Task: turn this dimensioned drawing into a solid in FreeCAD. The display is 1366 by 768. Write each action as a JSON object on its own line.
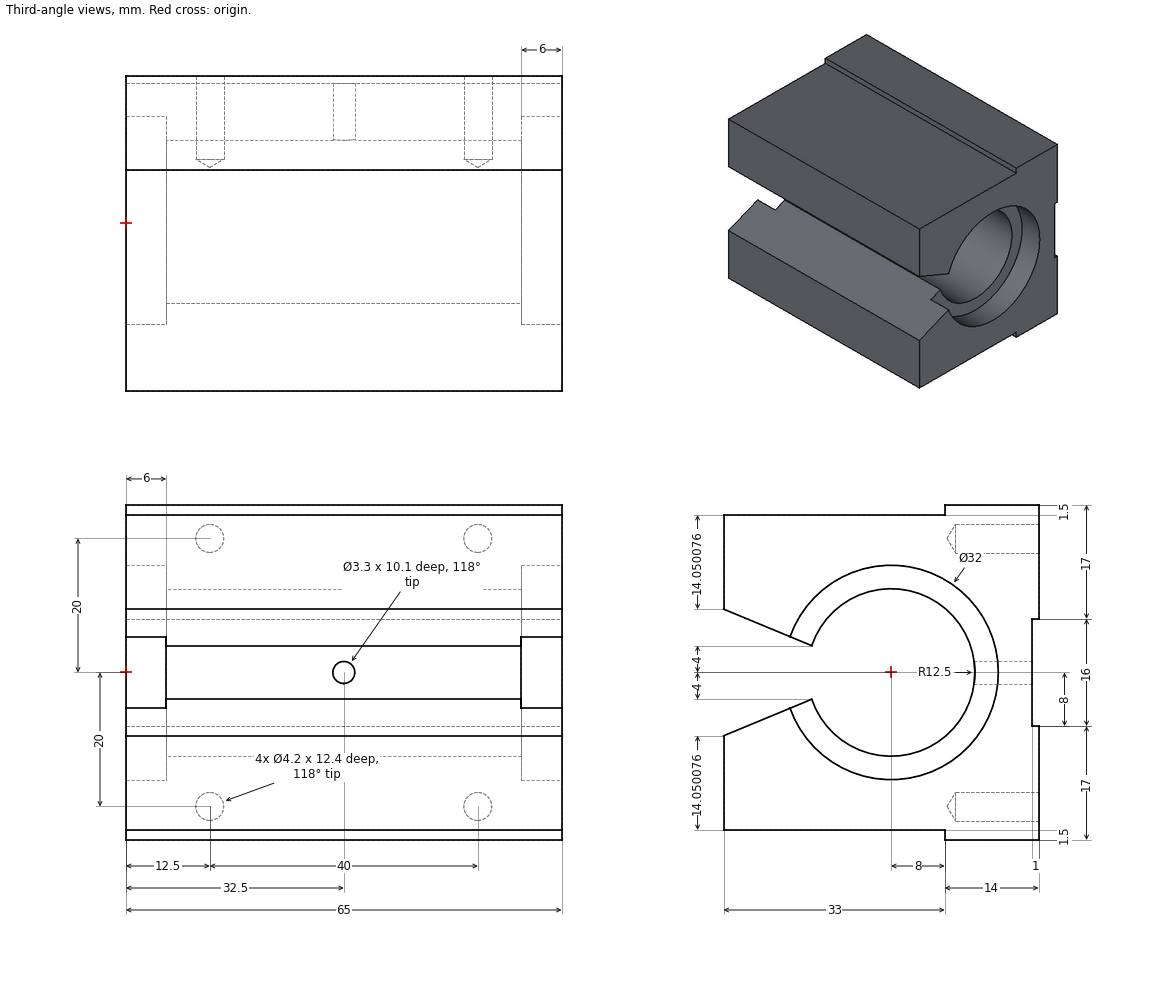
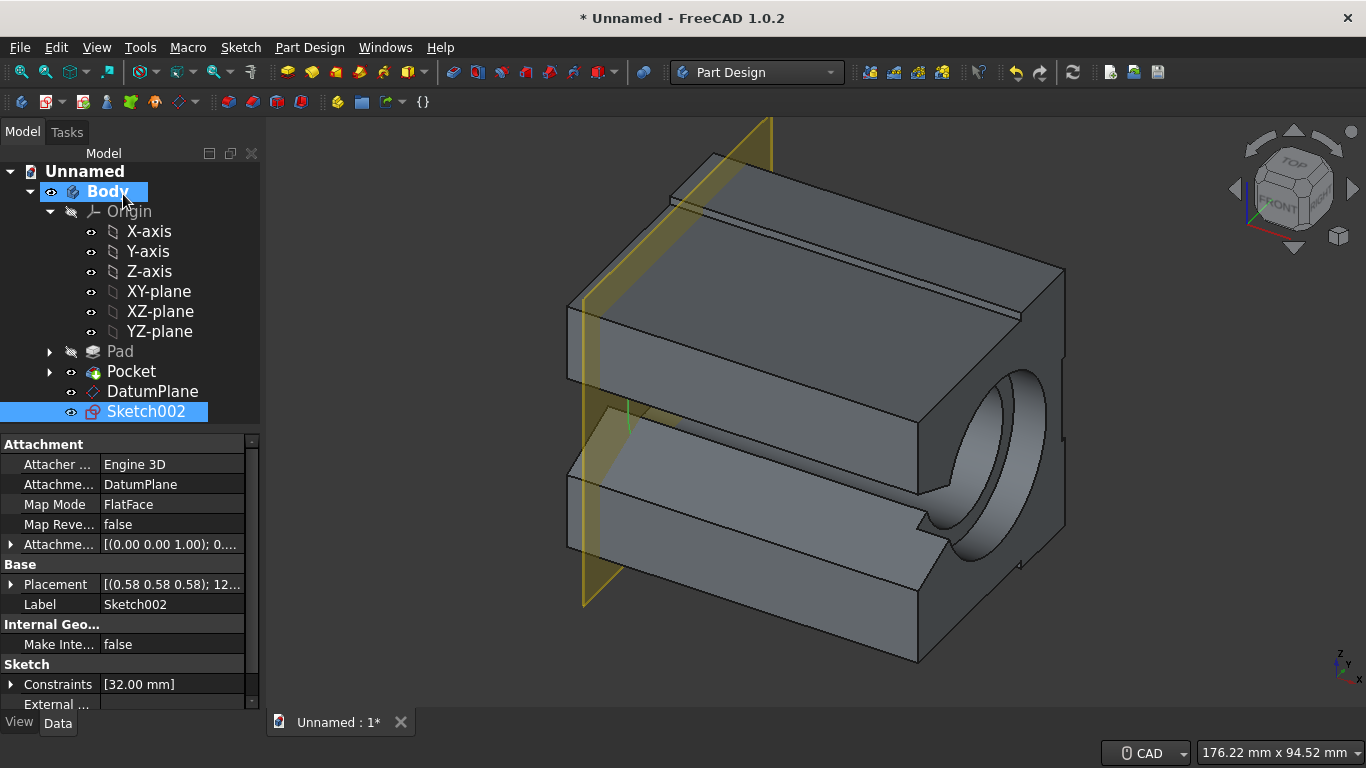
{"action": "left_click", "coordinate": [454, 72]}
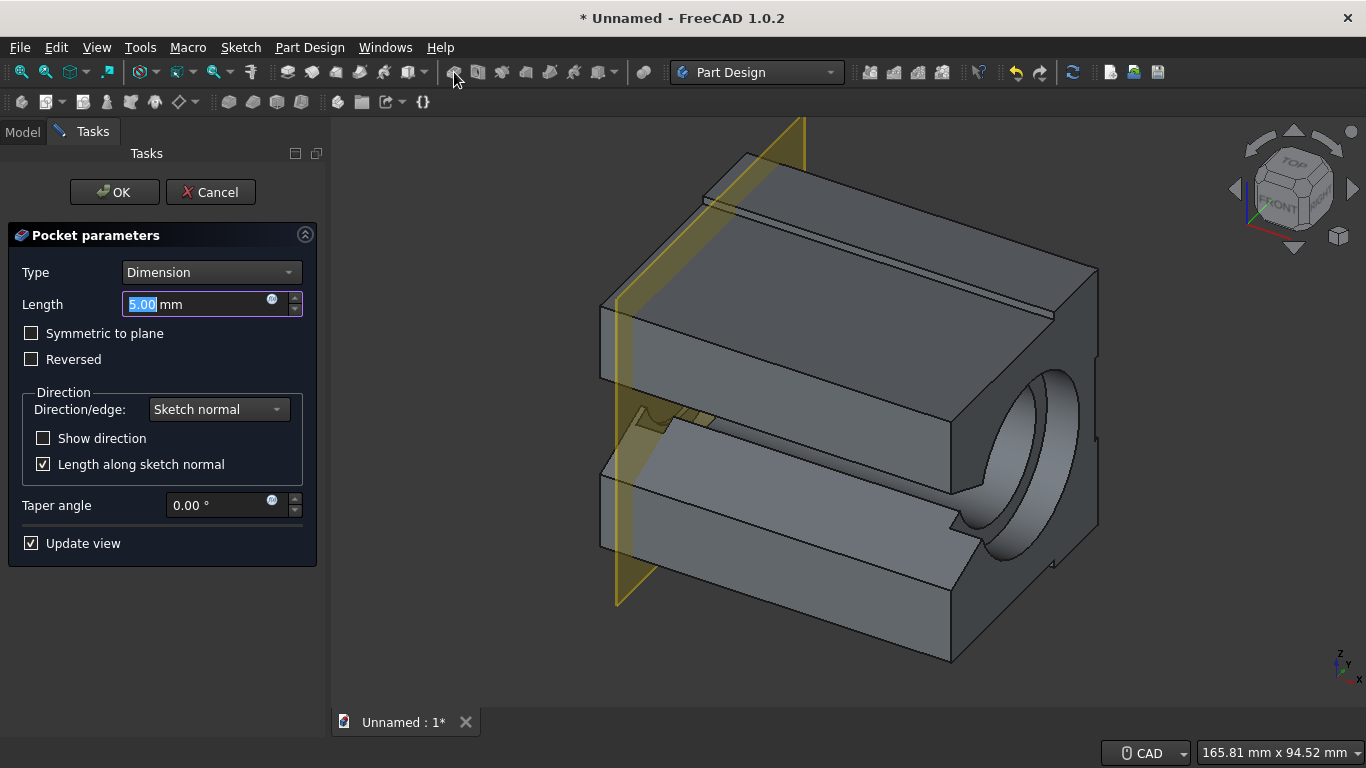
{"action": "type", "text": "6"}
{"action": "key", "text": "Tab"}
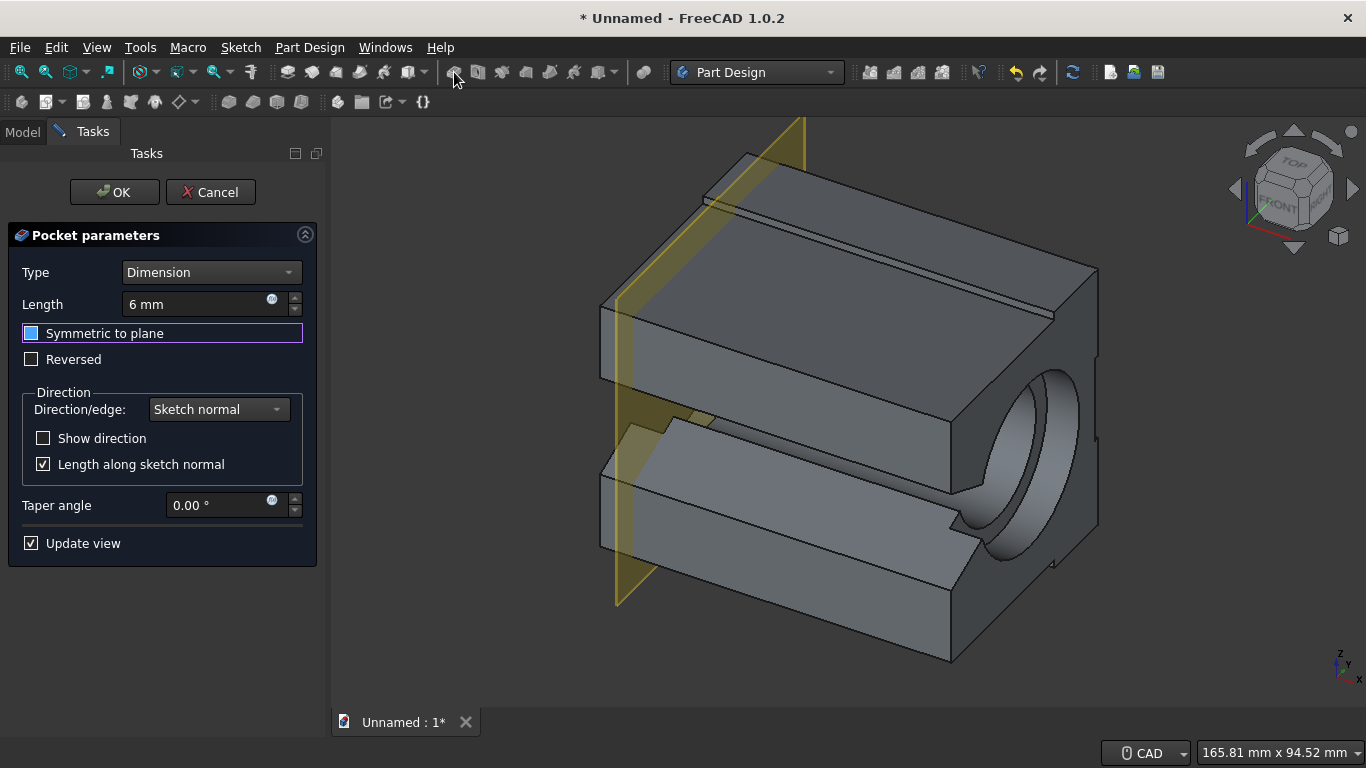
{"action": "left_click", "coordinate": [115, 192]}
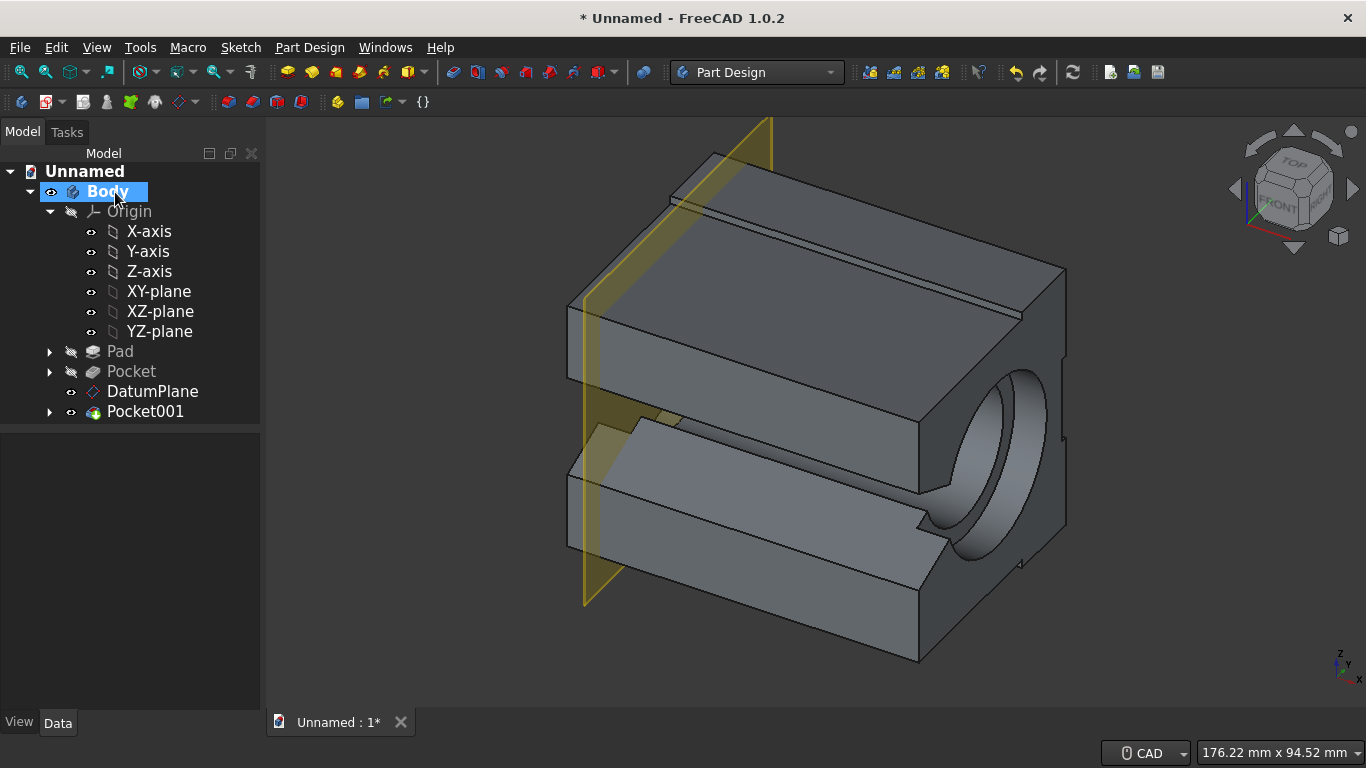
{"action": "left_click", "coordinate": [116, 392]}
{"action": "key", "text": "space"}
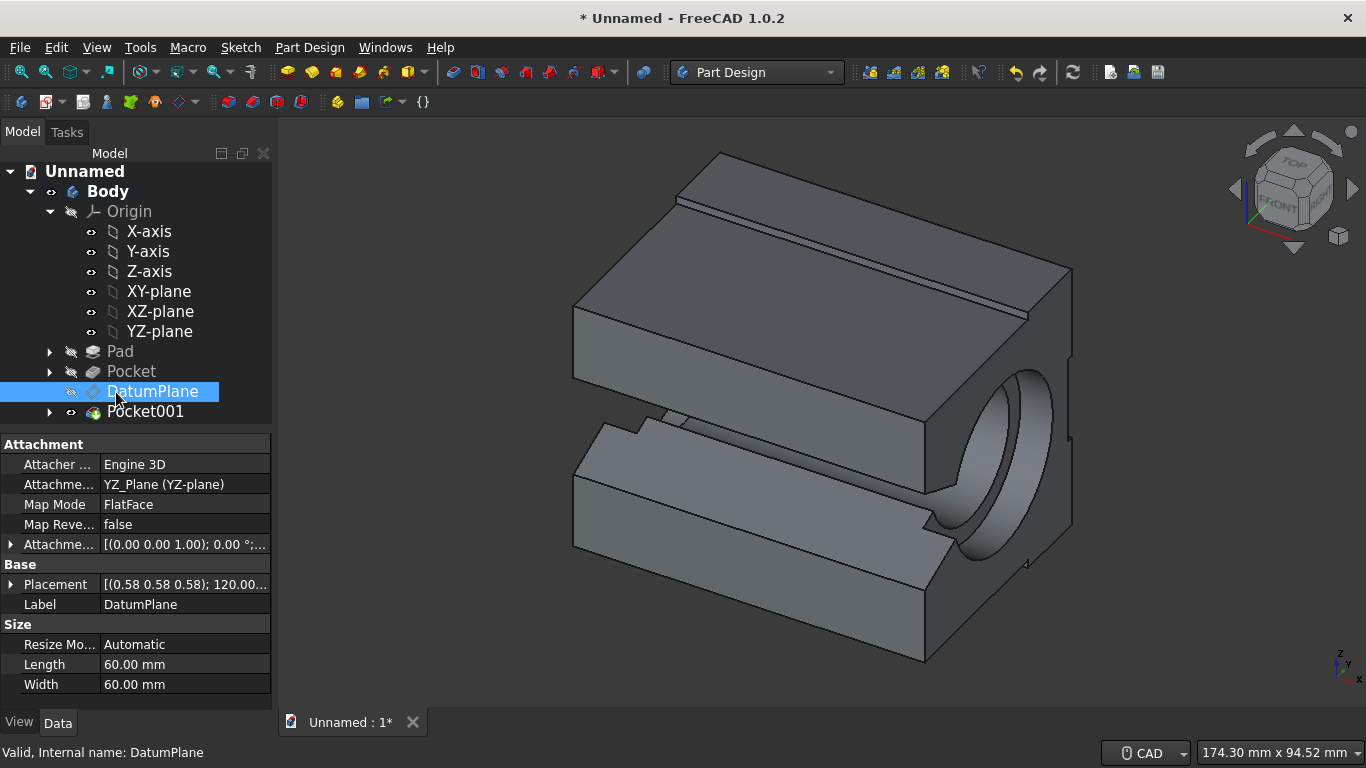
{"action": "key", "text": "4"}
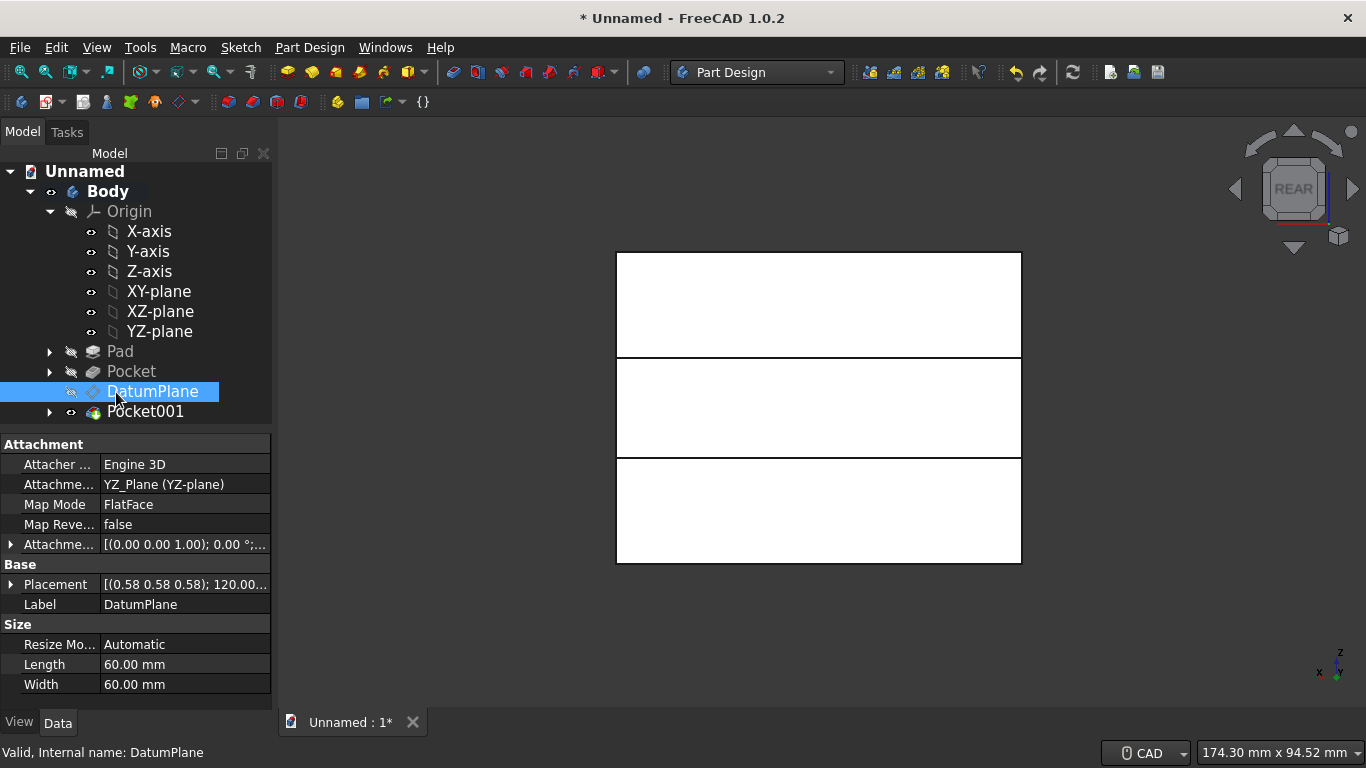
{"action": "left_click", "coordinate": [761, 304]}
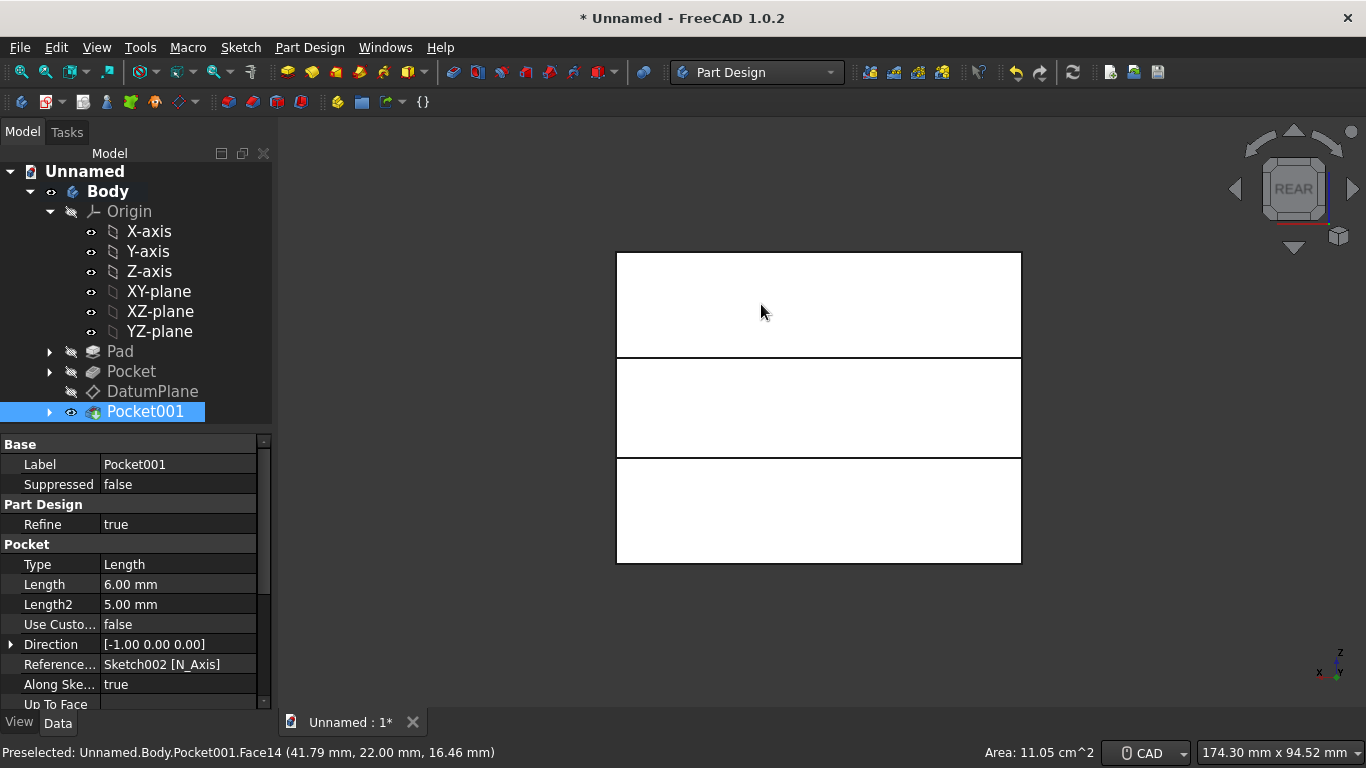
{"action": "left_click", "coordinate": [46, 102]}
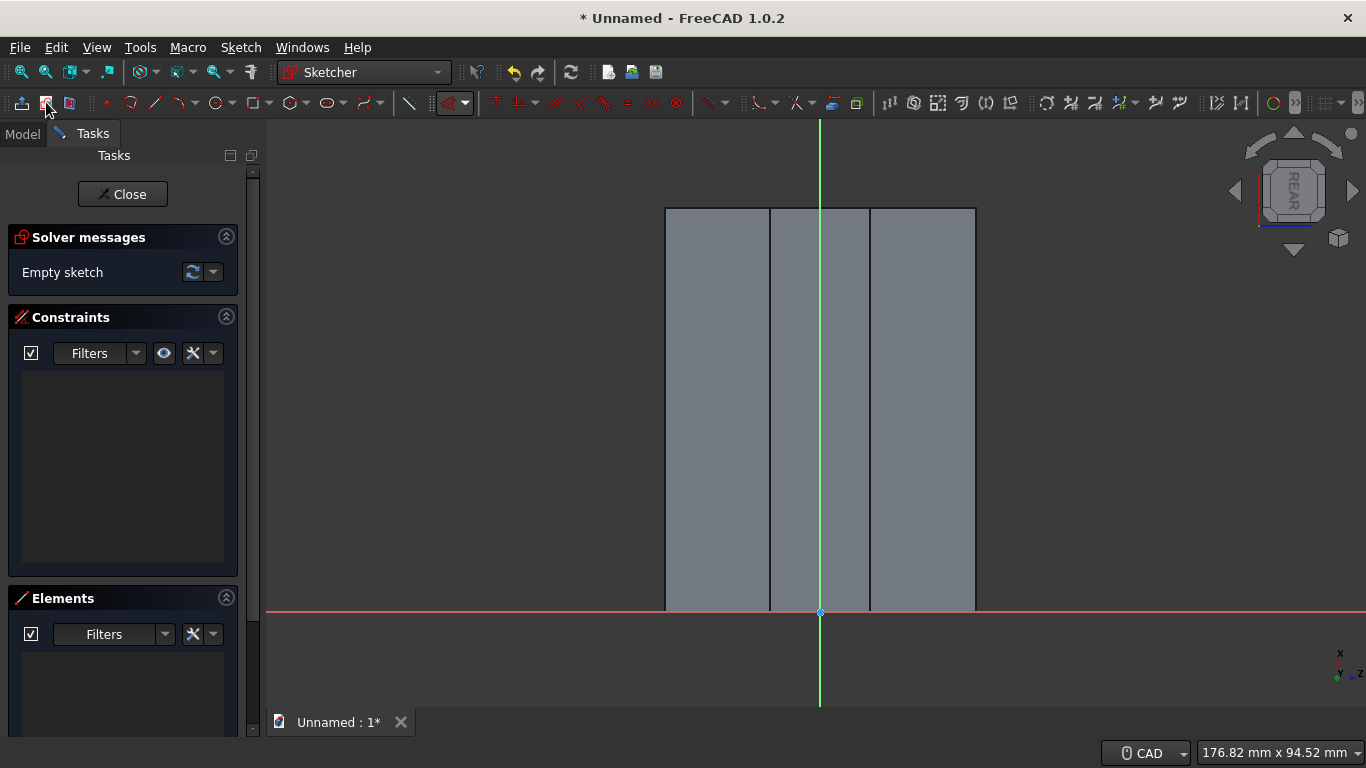
{"action": "key", "text": "g c"}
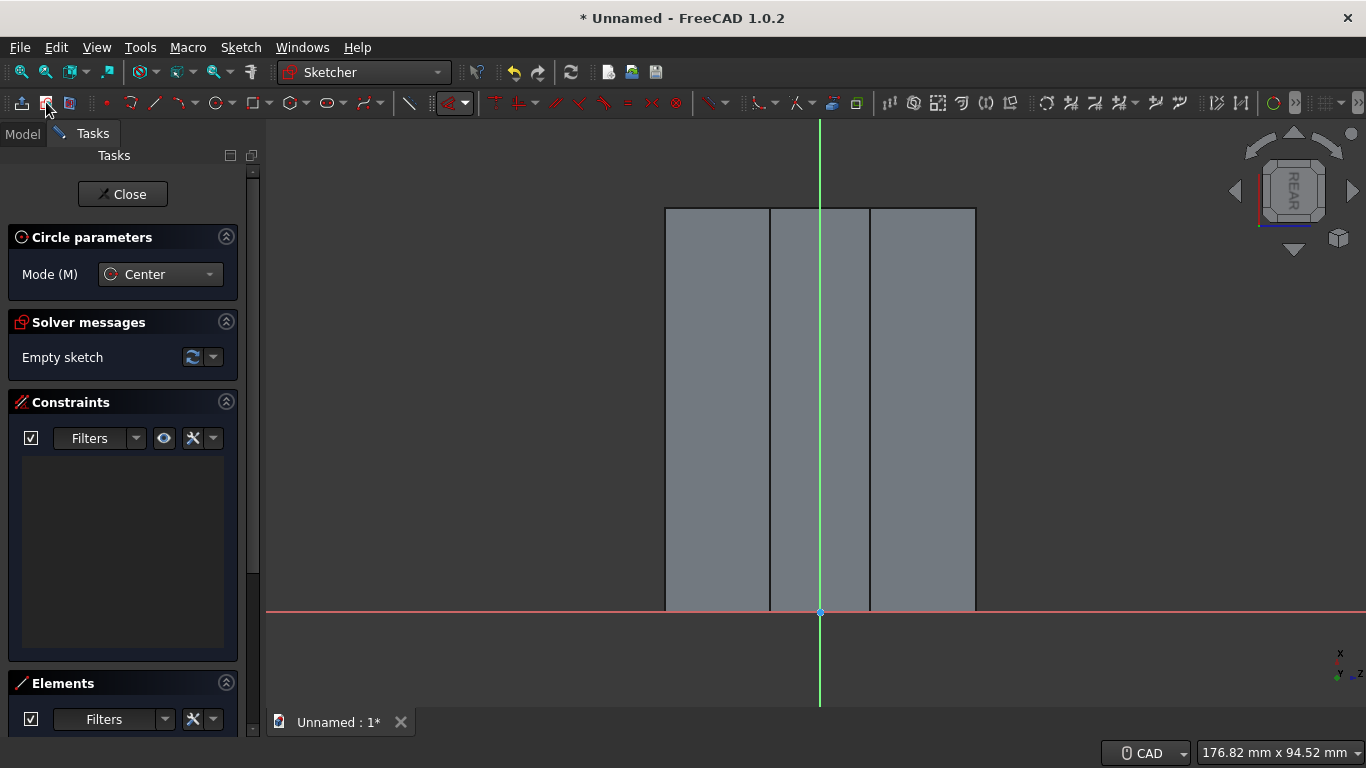
{"action": "scroll", "coordinate": [696, 534], "scroll_direction": "up", "scroll_amount": 3}